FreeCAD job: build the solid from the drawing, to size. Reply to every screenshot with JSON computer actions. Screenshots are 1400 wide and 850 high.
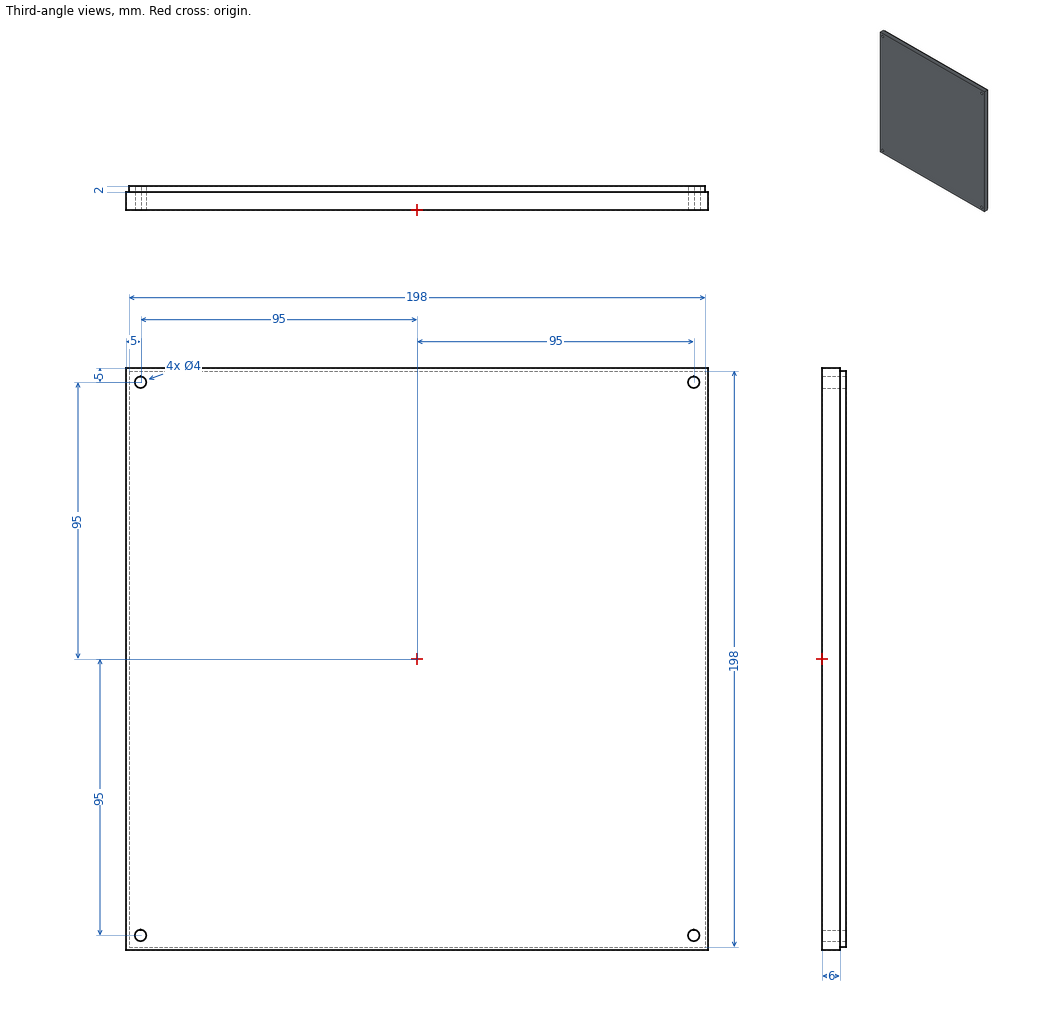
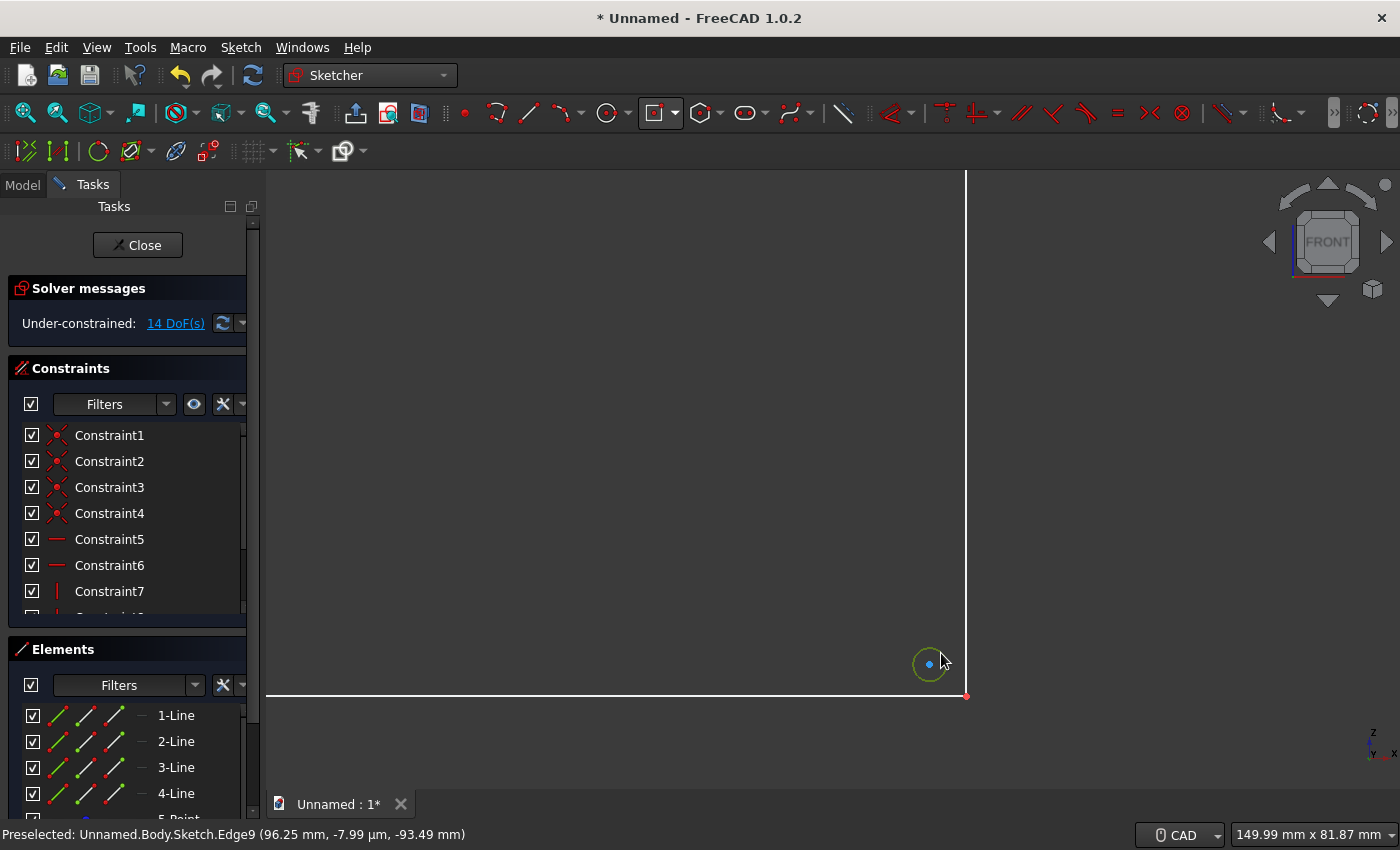
{"action": "key", "text": "e"}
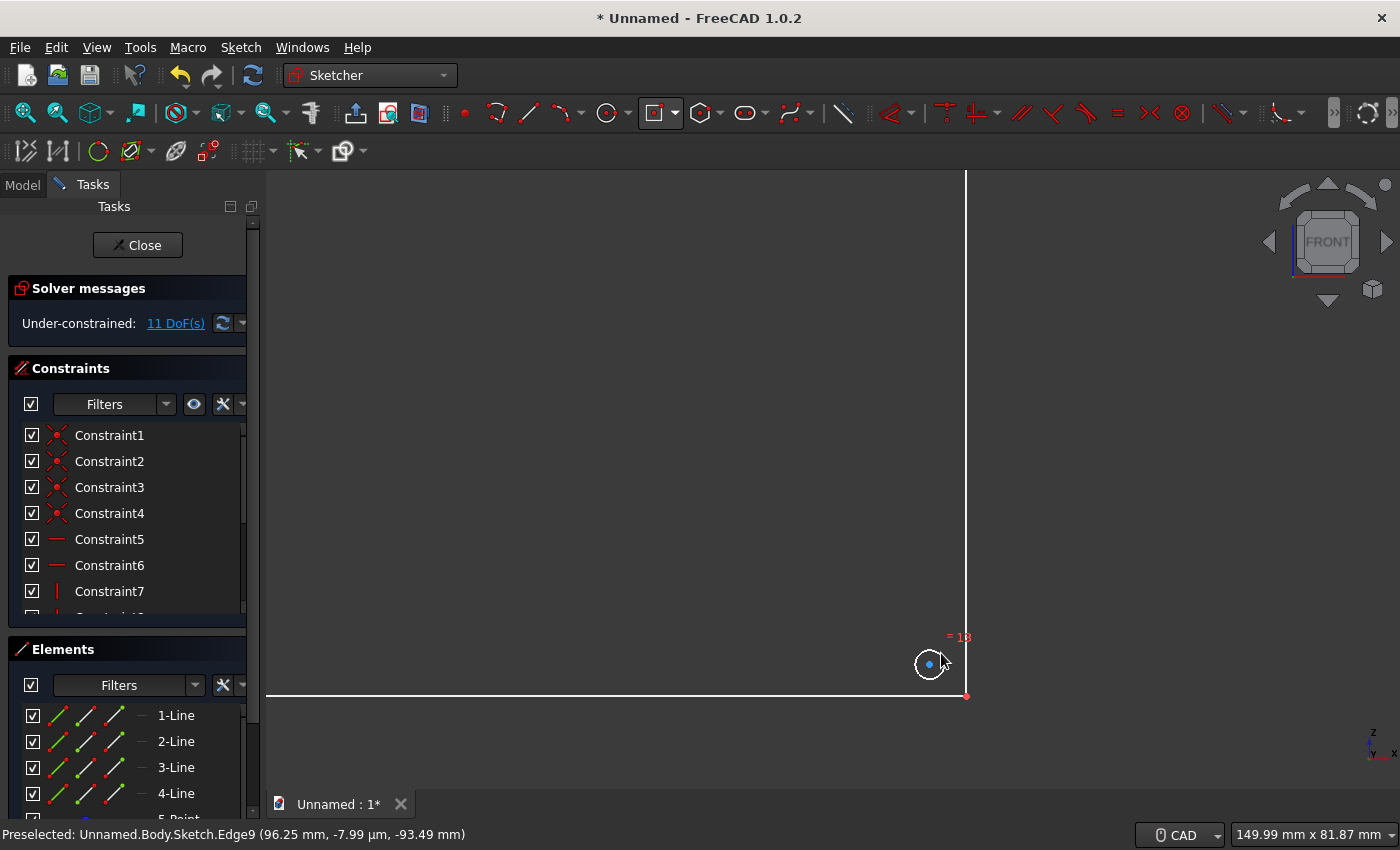
{"action": "scroll", "coordinate": [946, 655], "scroll_direction": "down", "scroll_amount": 7}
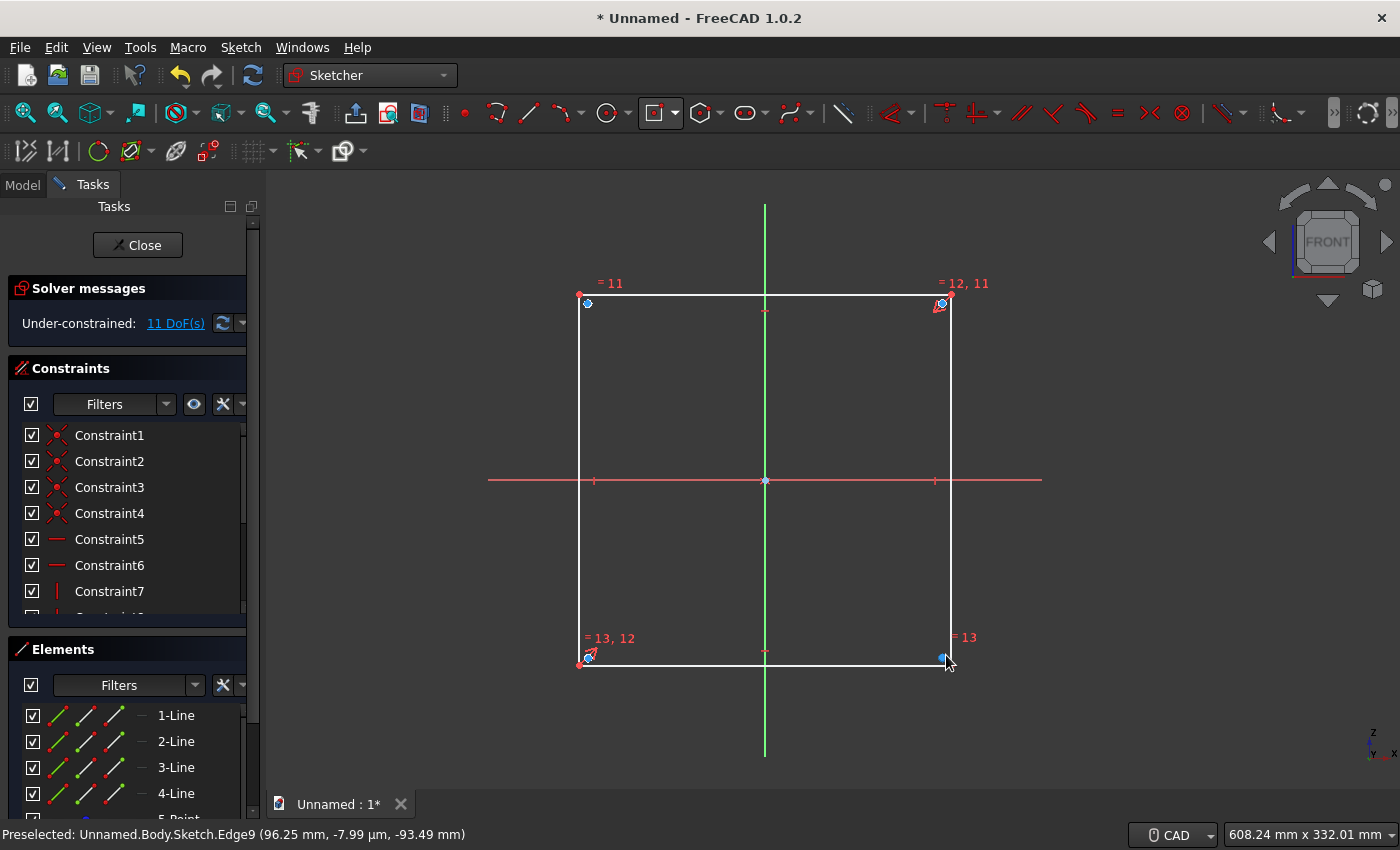
{"action": "left_click", "coordinate": [588, 304]}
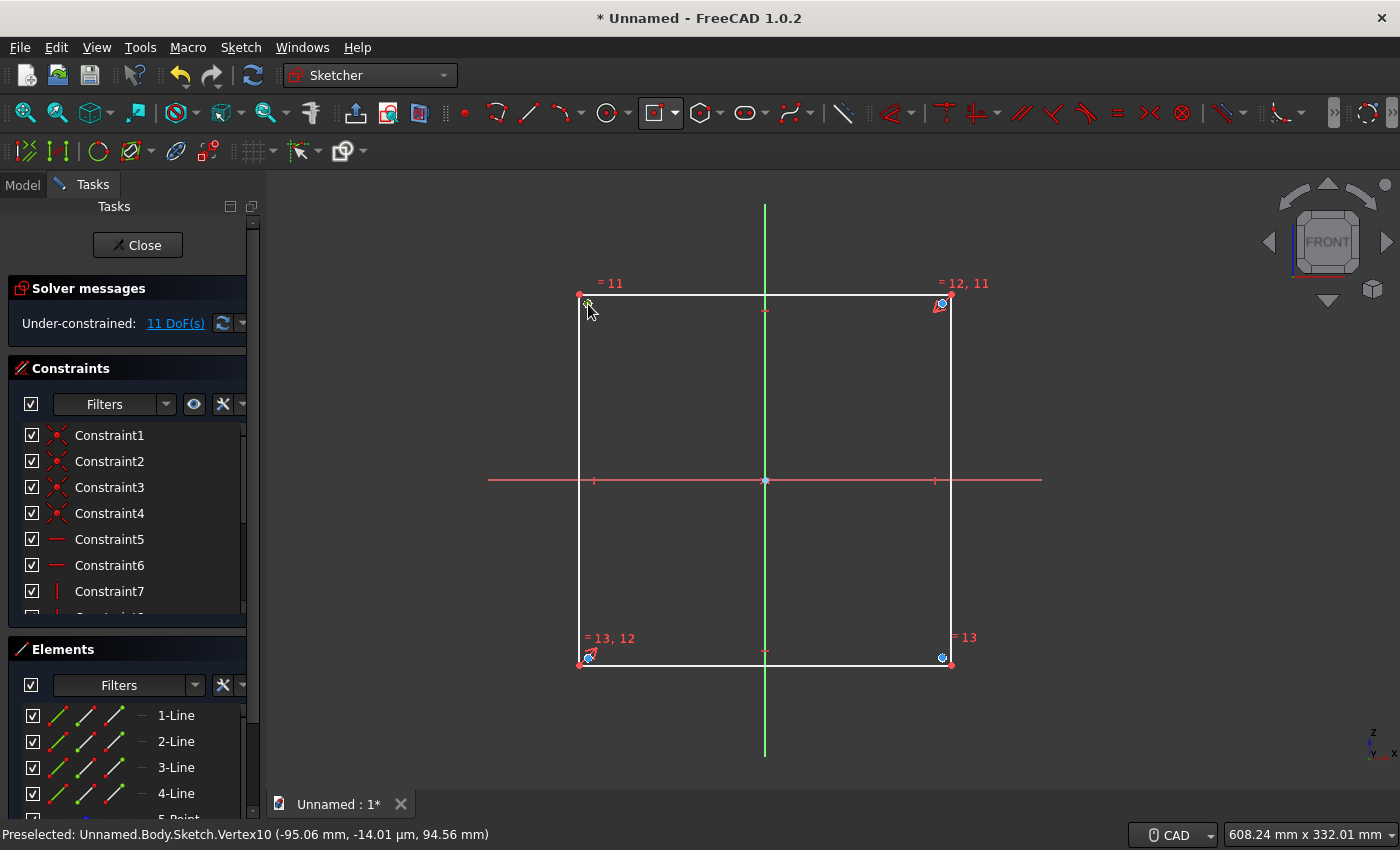
{"action": "left_click", "coordinate": [942, 304]}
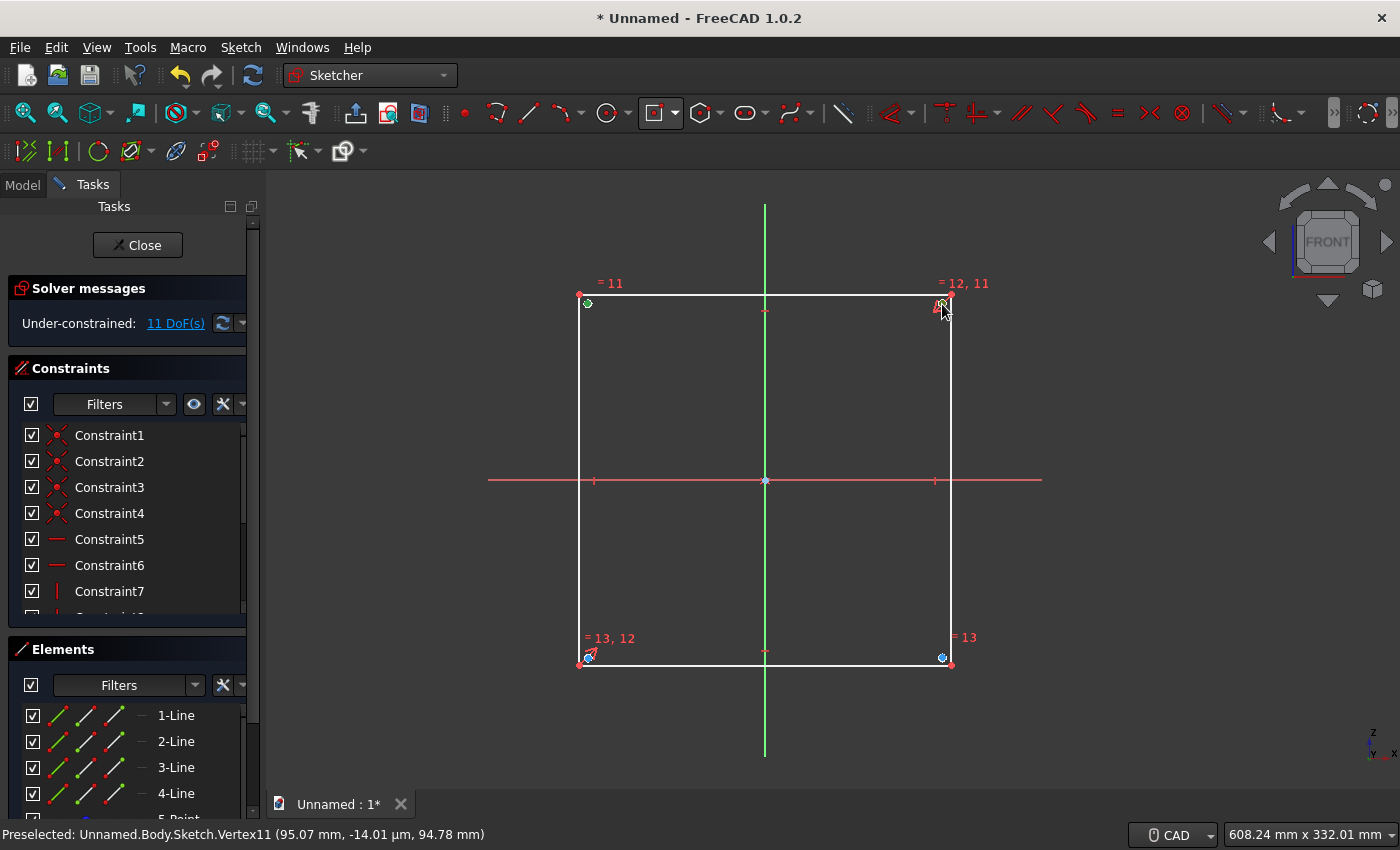
{"action": "key", "text": "h"}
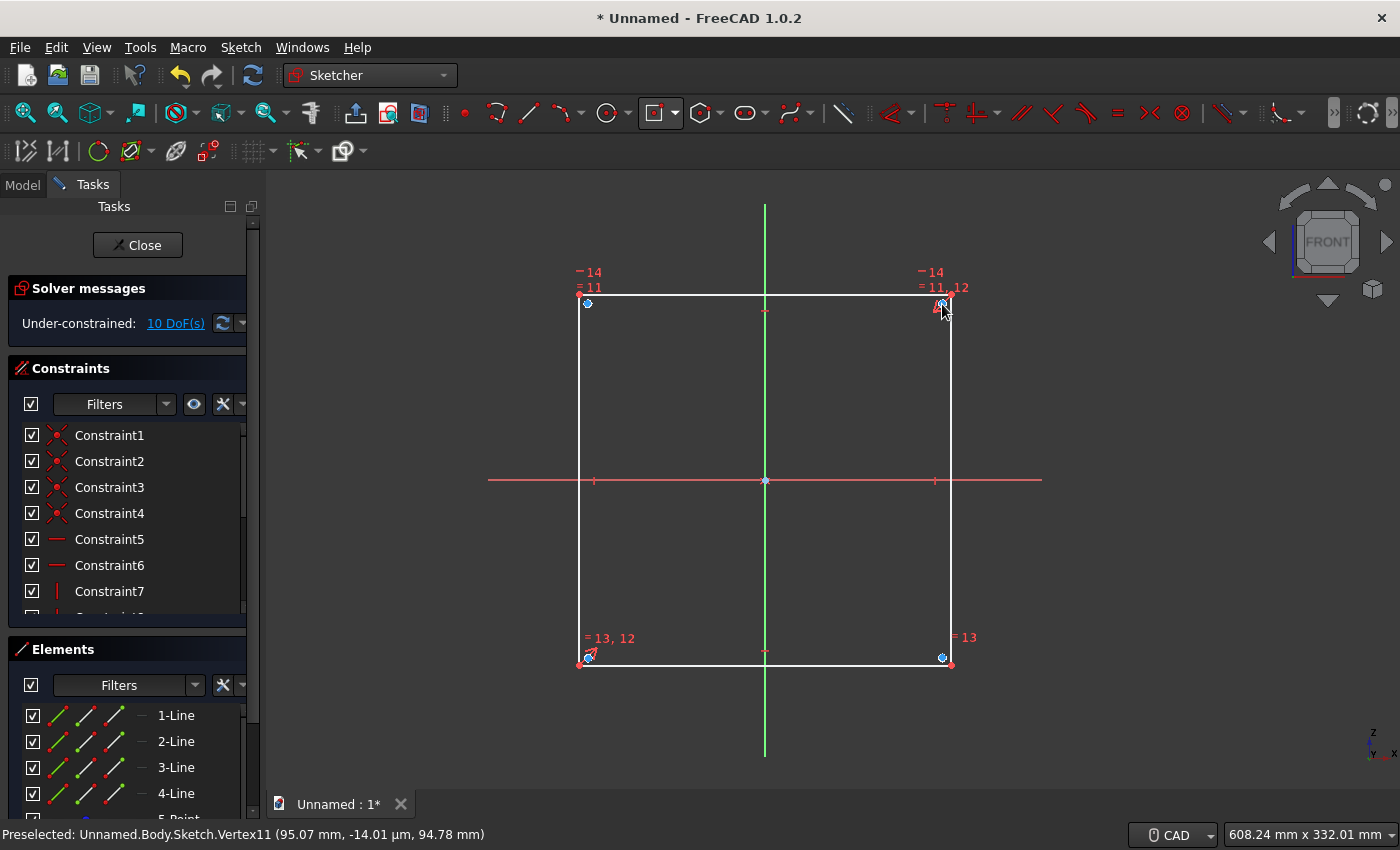
{"action": "left_click", "coordinate": [588, 304]}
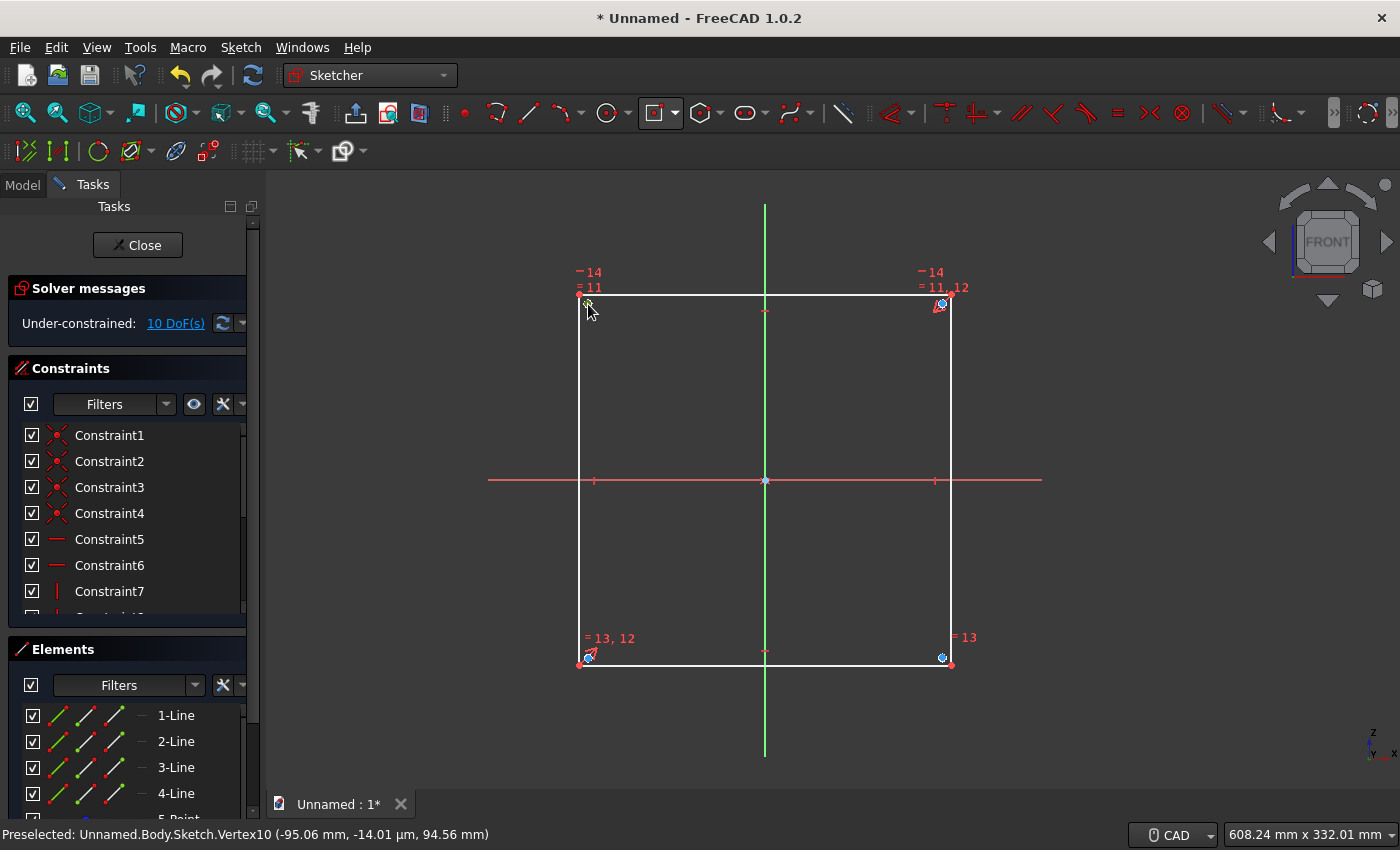
{"action": "left_click", "coordinate": [588, 658]}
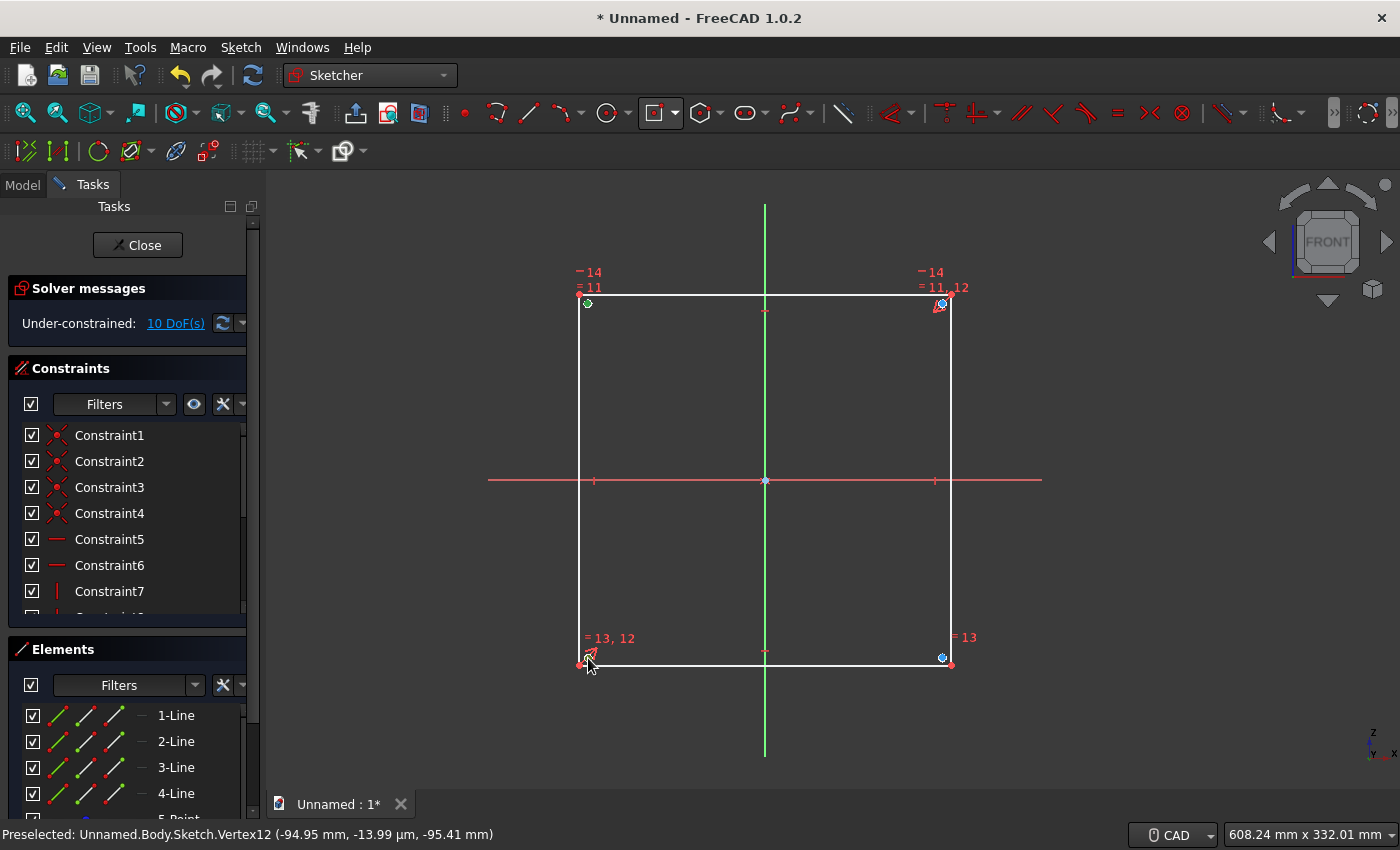
{"action": "key", "text": "v"}